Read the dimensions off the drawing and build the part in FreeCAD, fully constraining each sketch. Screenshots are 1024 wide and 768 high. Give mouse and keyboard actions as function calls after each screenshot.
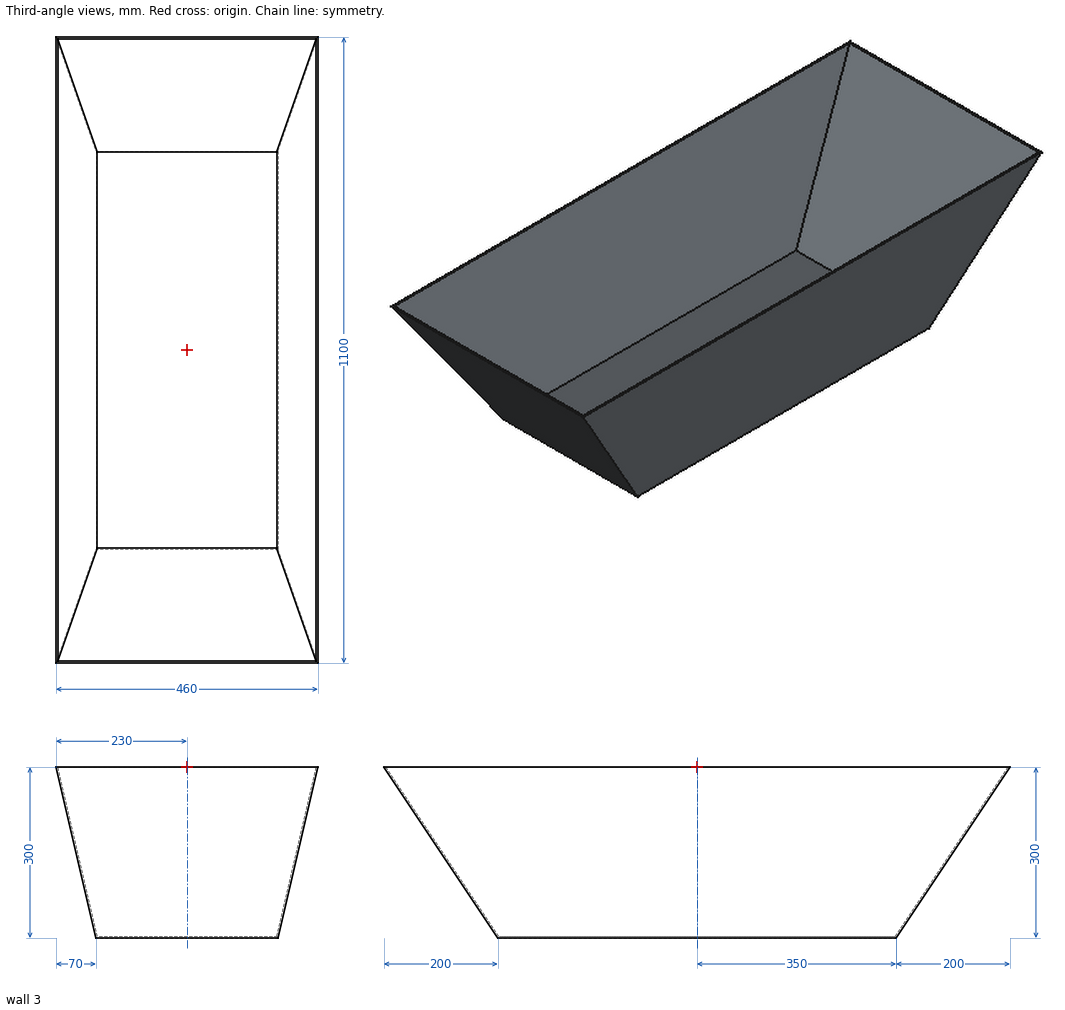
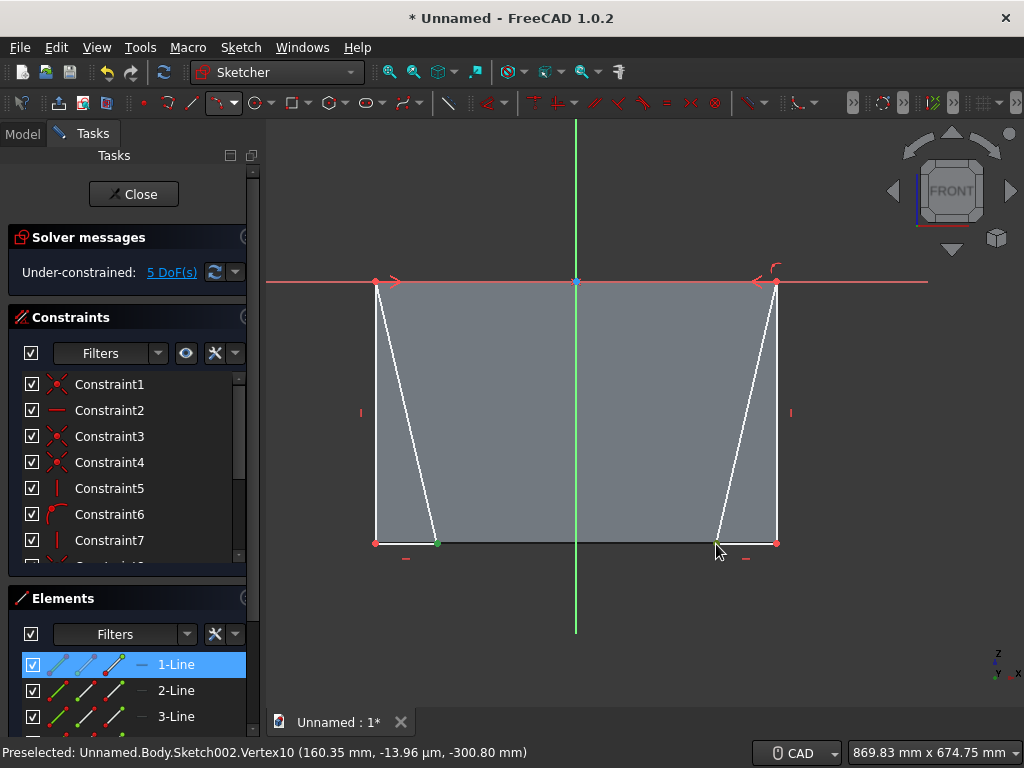
click(576, 603)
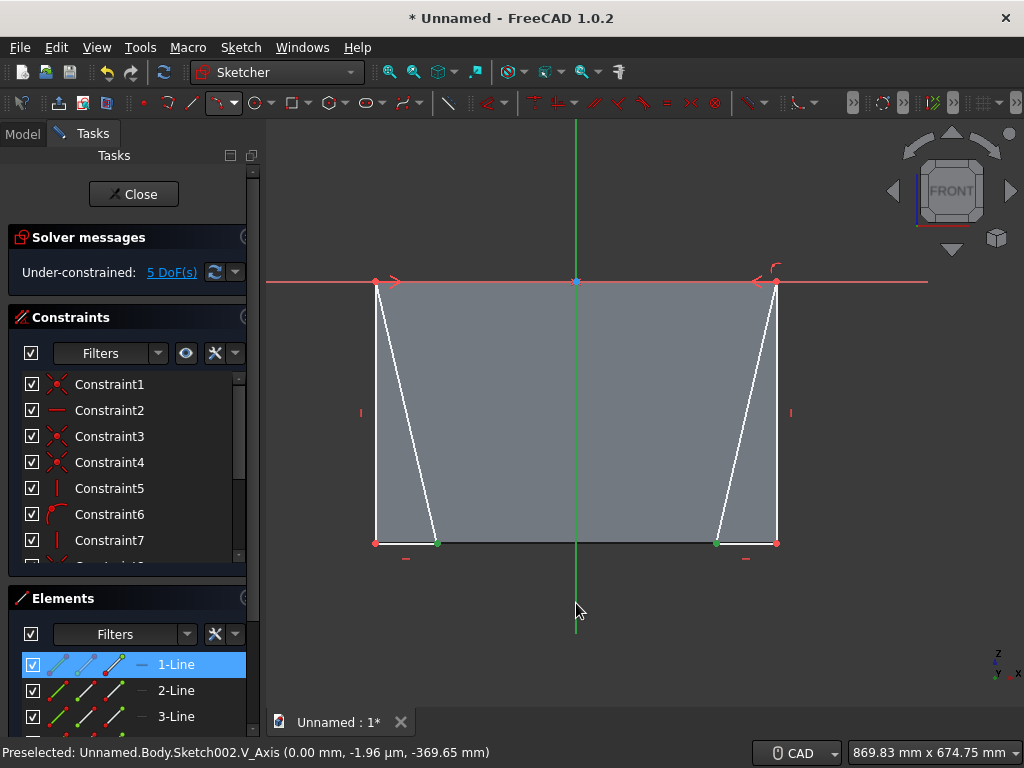
click(692, 104)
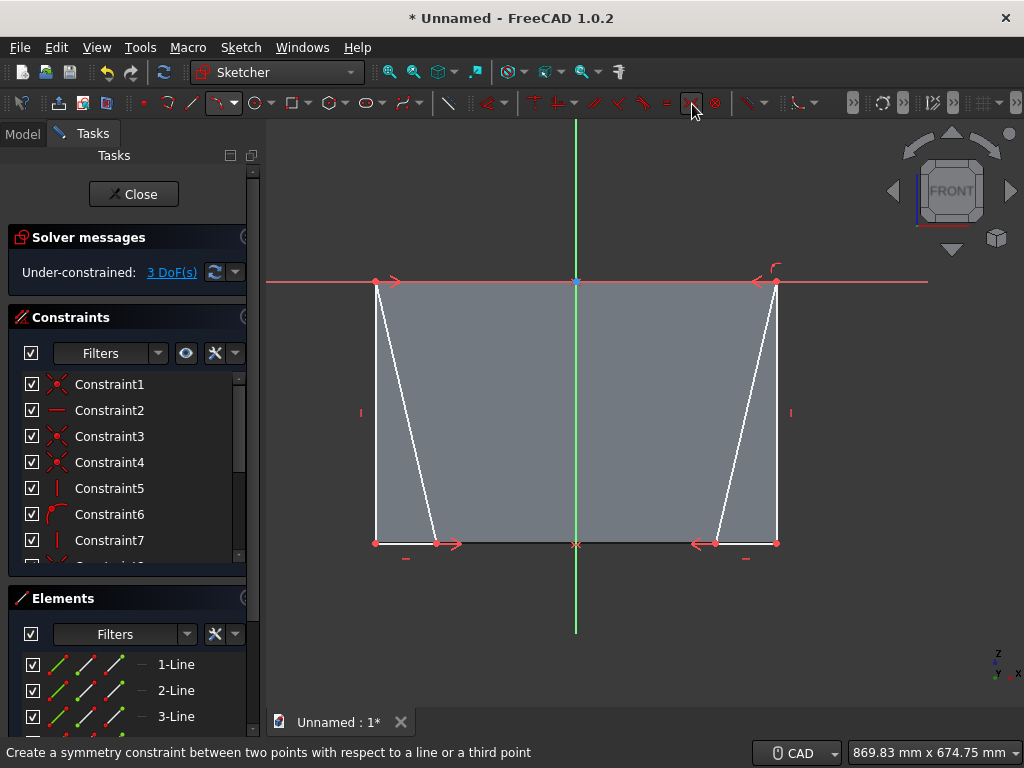
click(488, 104)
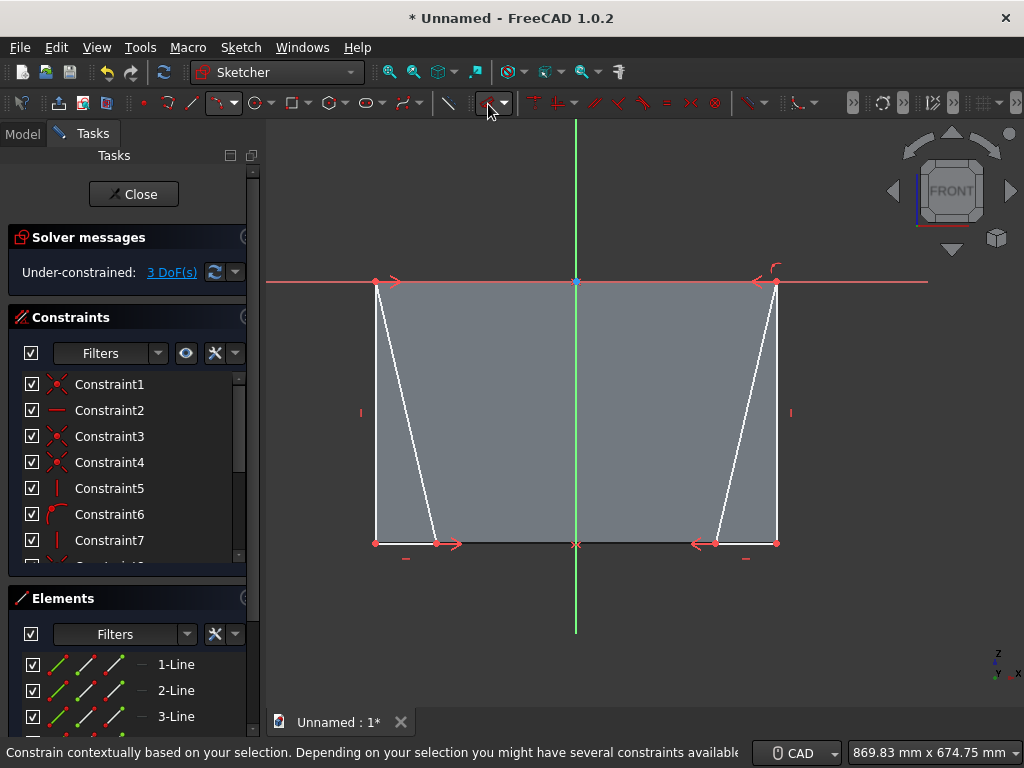
click(419, 544)
click(406, 578)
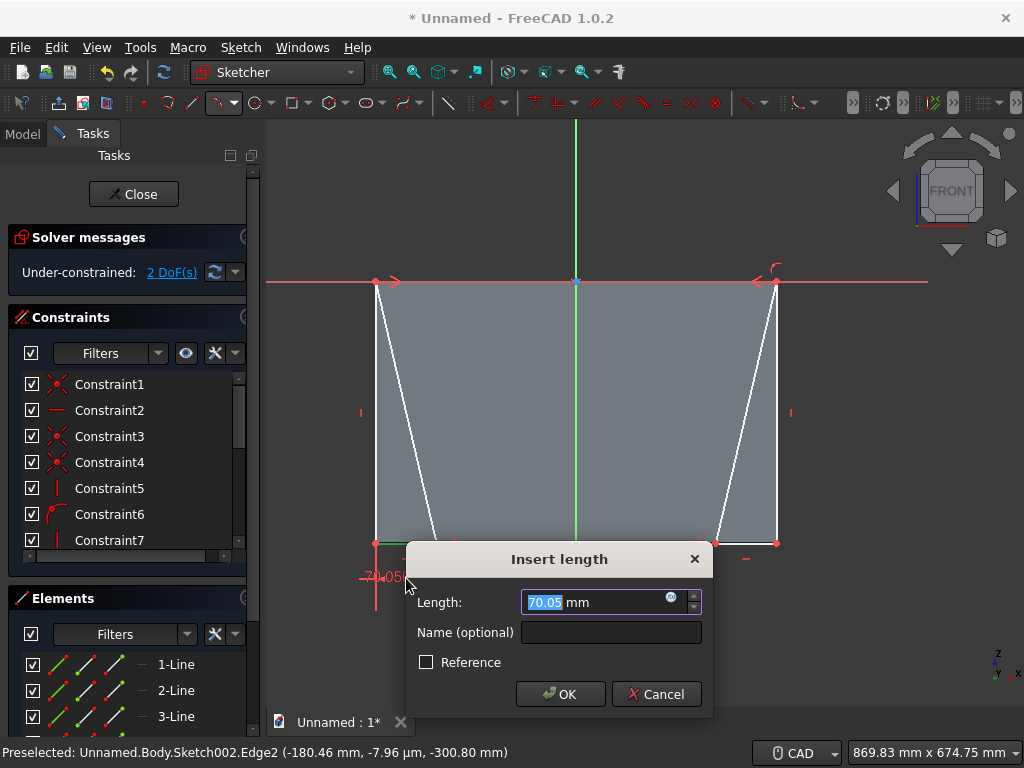
text(70)
key(Return)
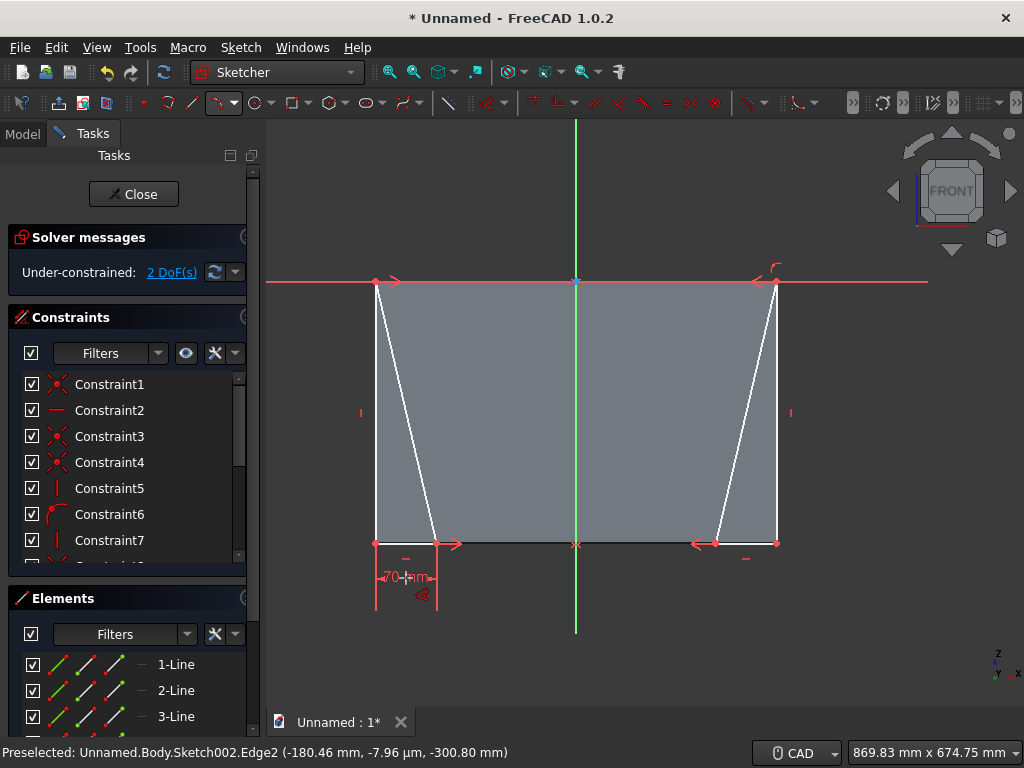
click(376, 465)
click(342, 413)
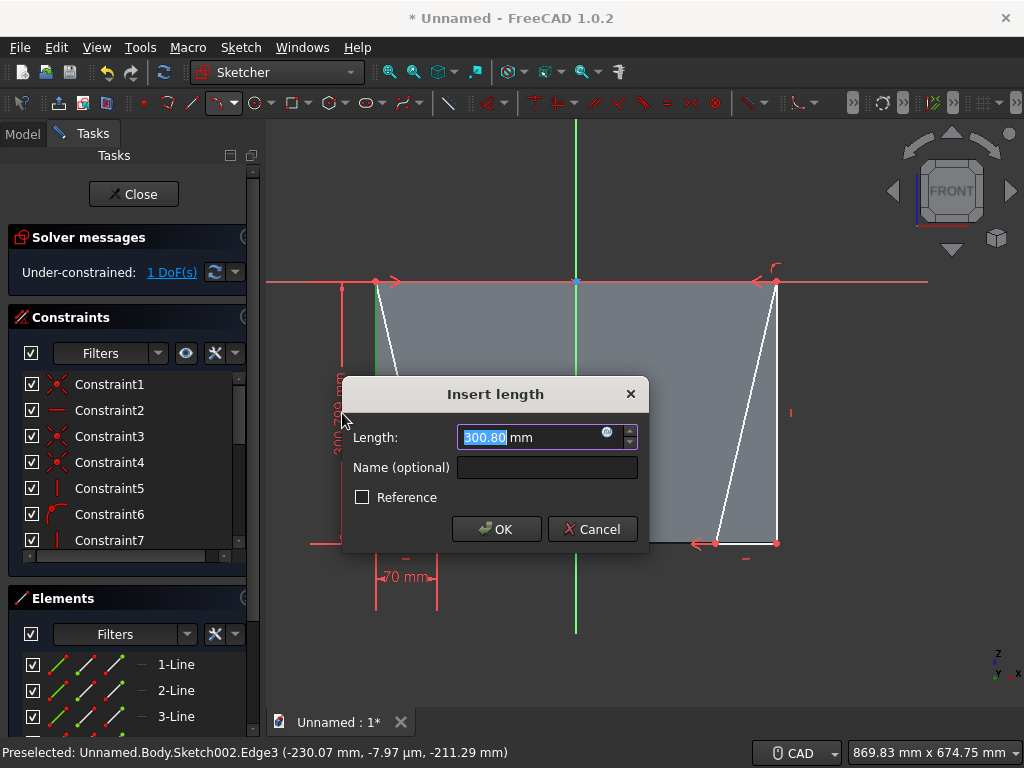
text(300)
key(Return)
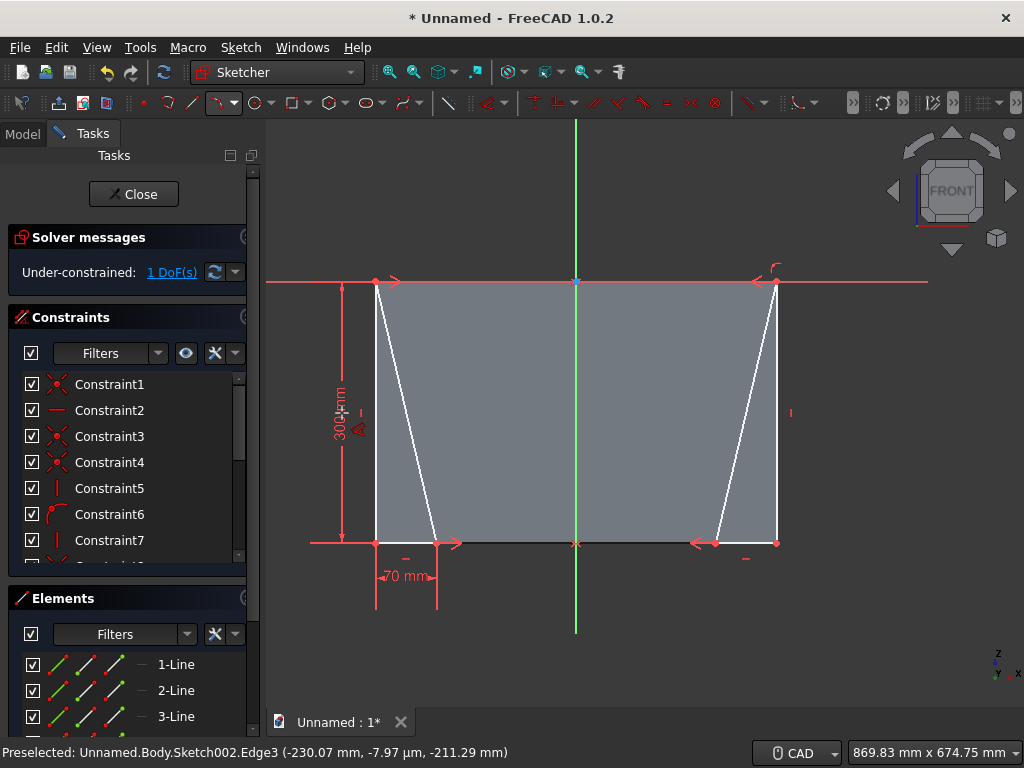
click(376, 282)
click(476, 248)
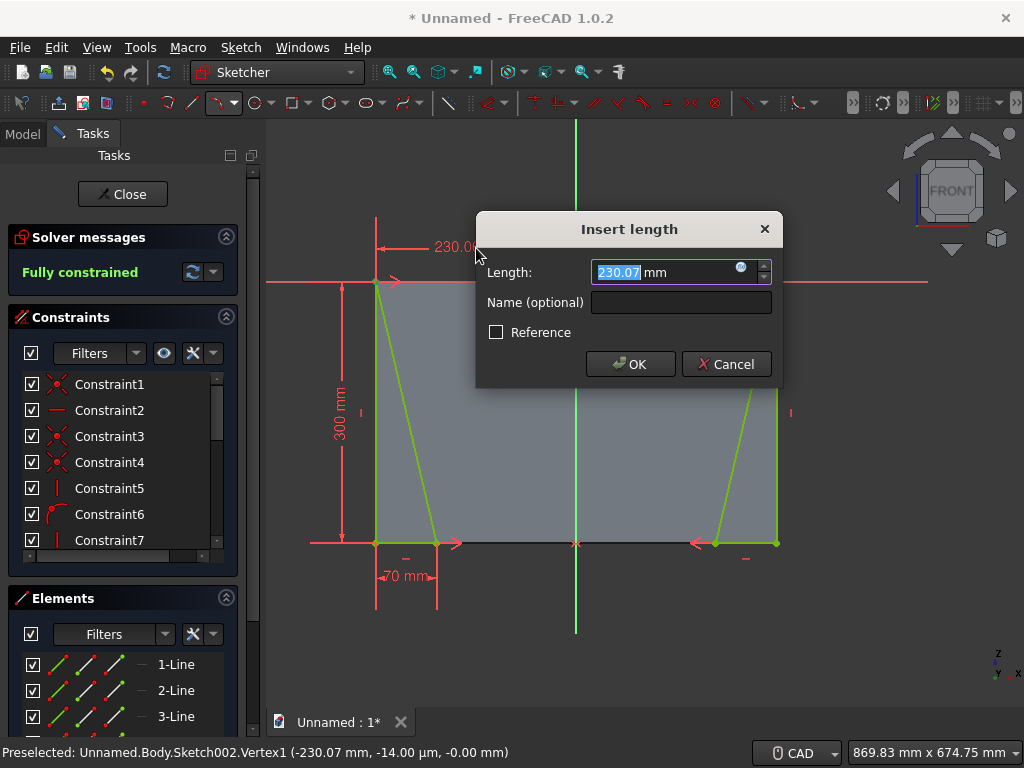
text(230)
key(Return)
key(Escape)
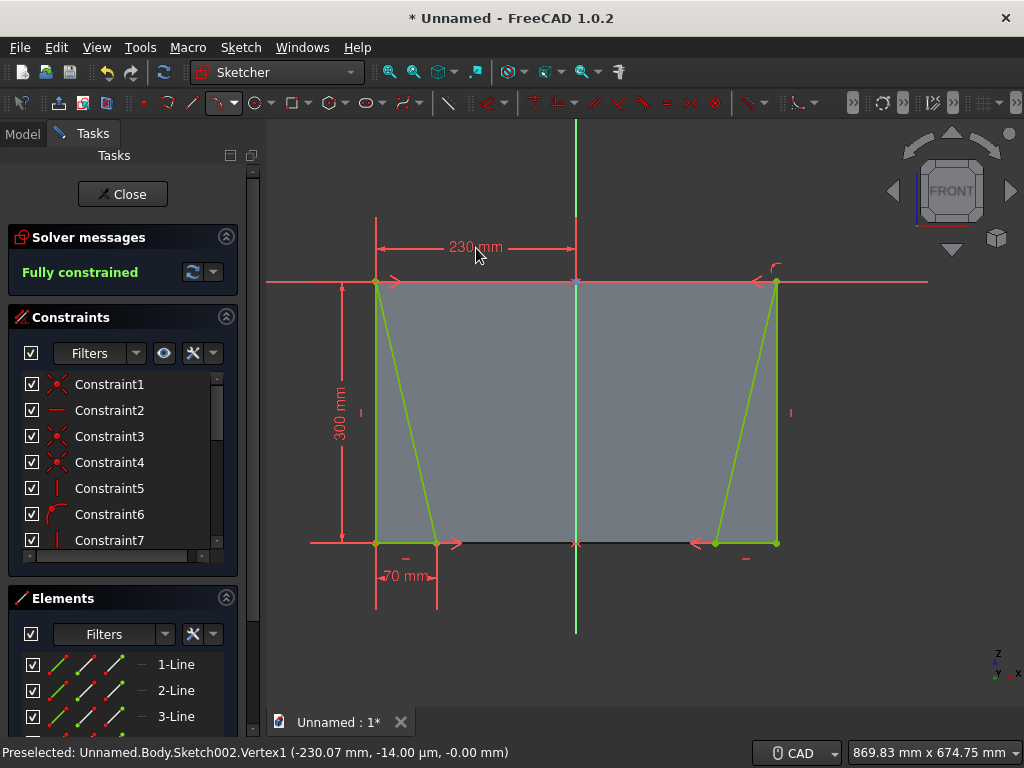
click(123, 194)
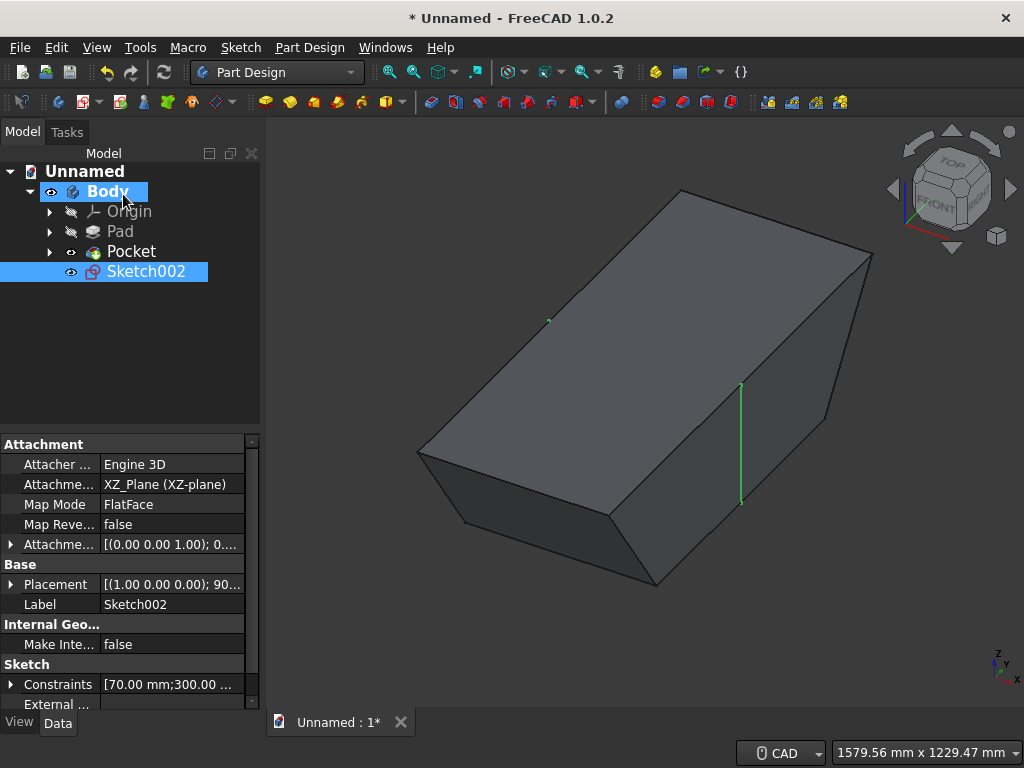
click(432, 102)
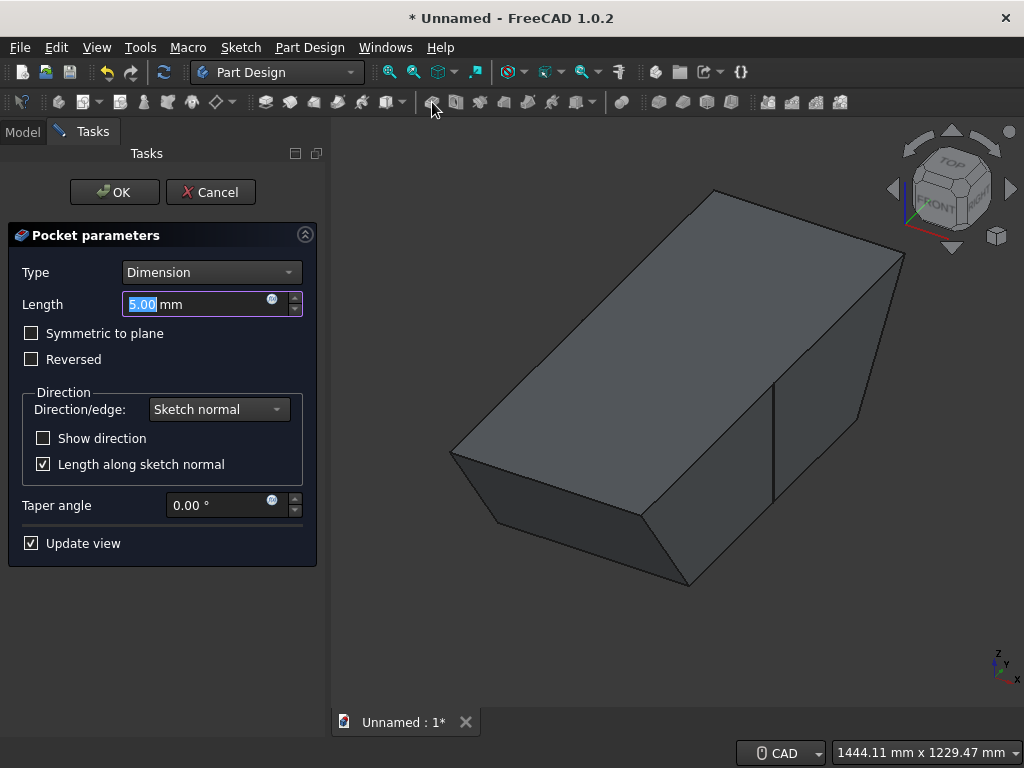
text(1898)
key(Tab)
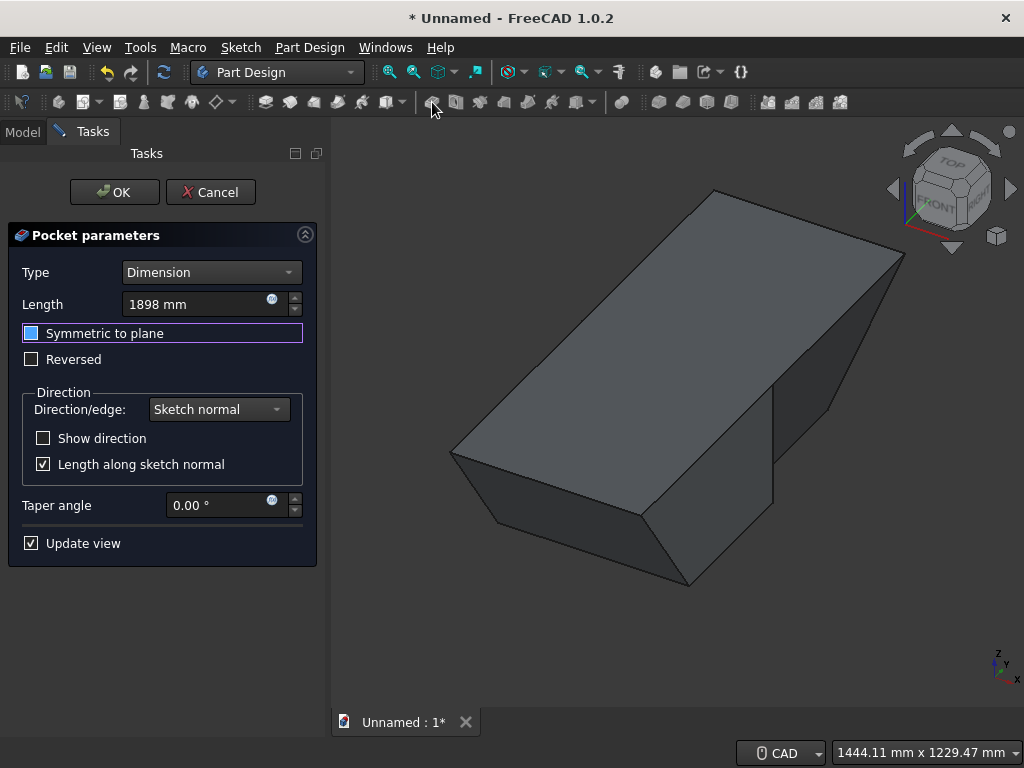
click(30, 333)